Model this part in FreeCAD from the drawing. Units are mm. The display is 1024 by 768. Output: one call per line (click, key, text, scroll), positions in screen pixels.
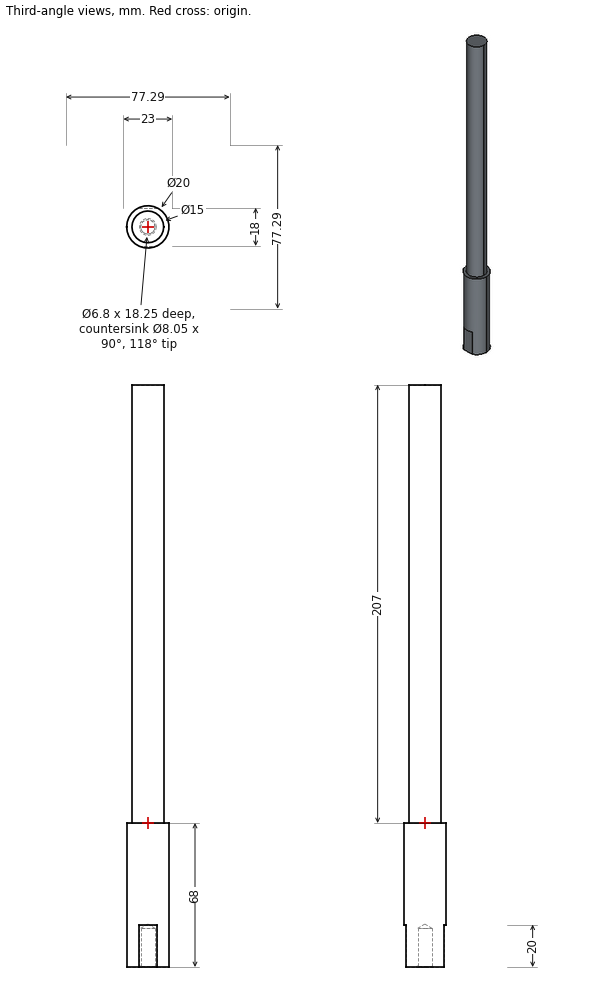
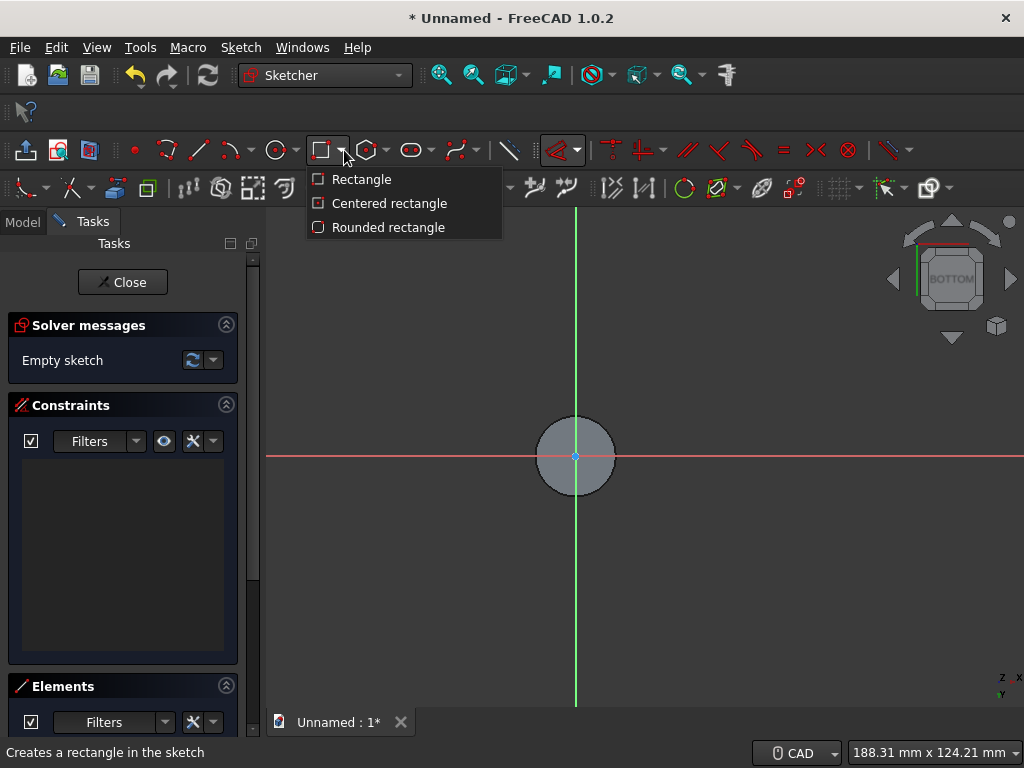
click(404, 203)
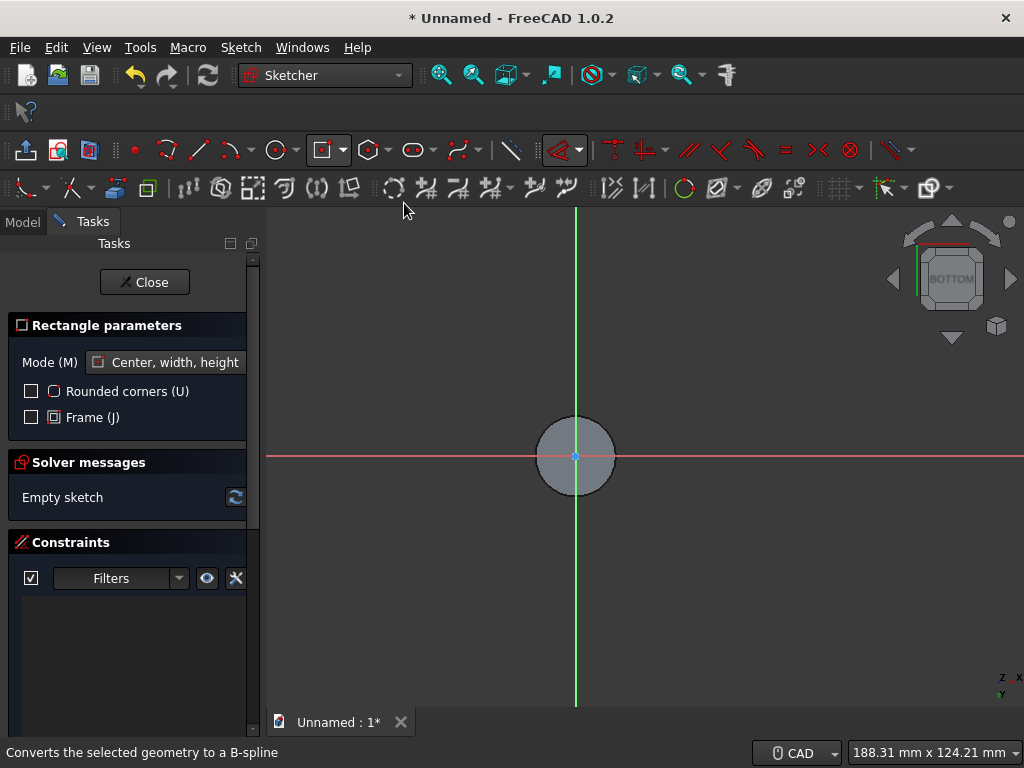
click(576, 456)
click(731, 301)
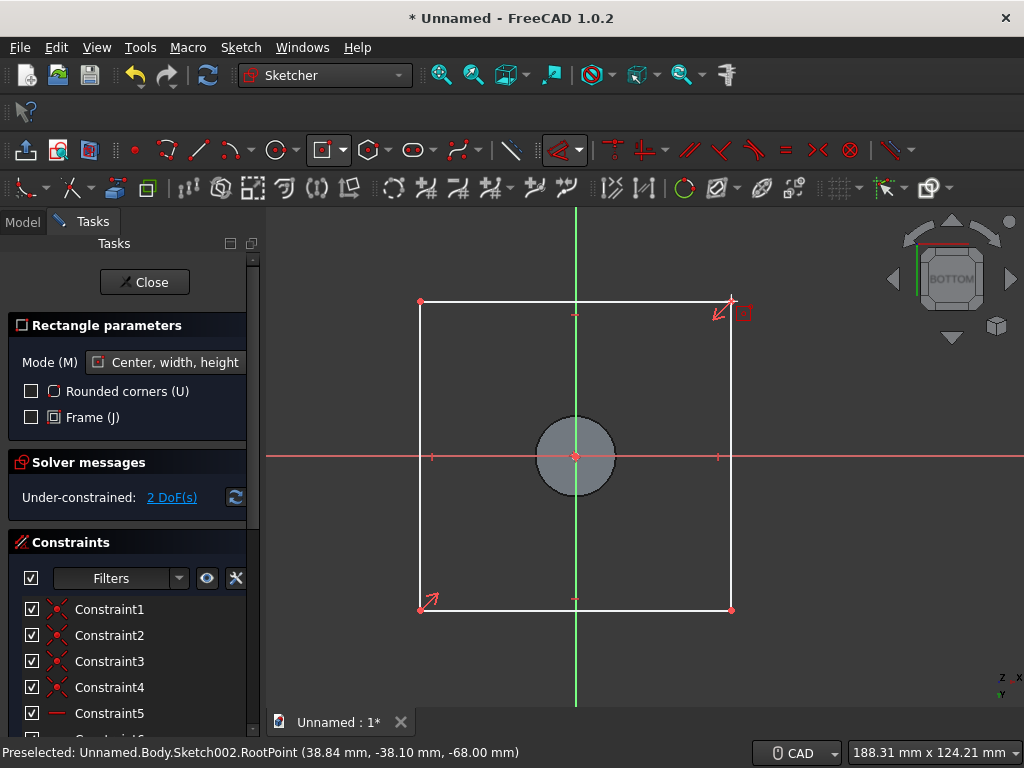
click(576, 456)
click(622, 420)
key(Escape)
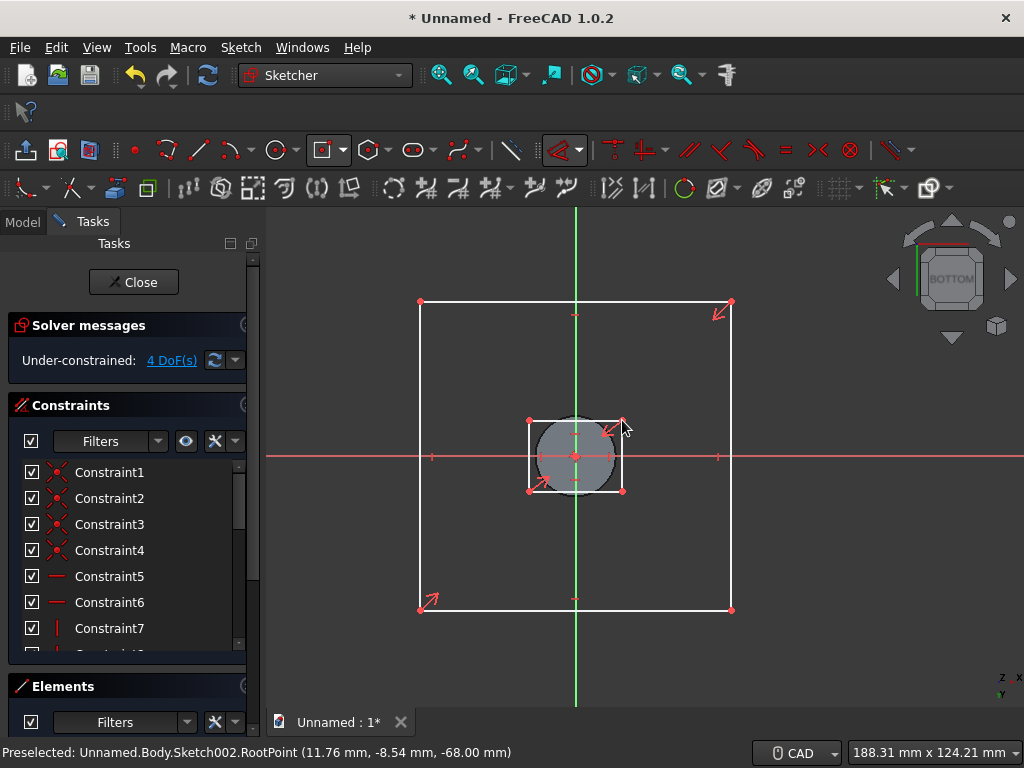
click(557, 492)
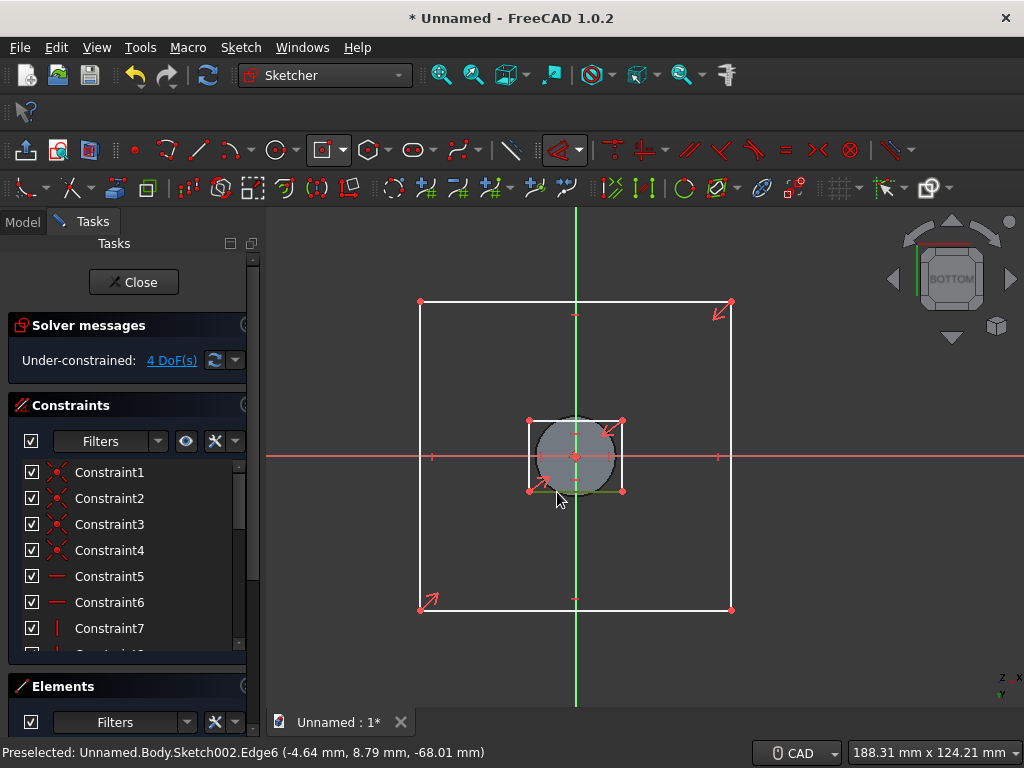
key(l)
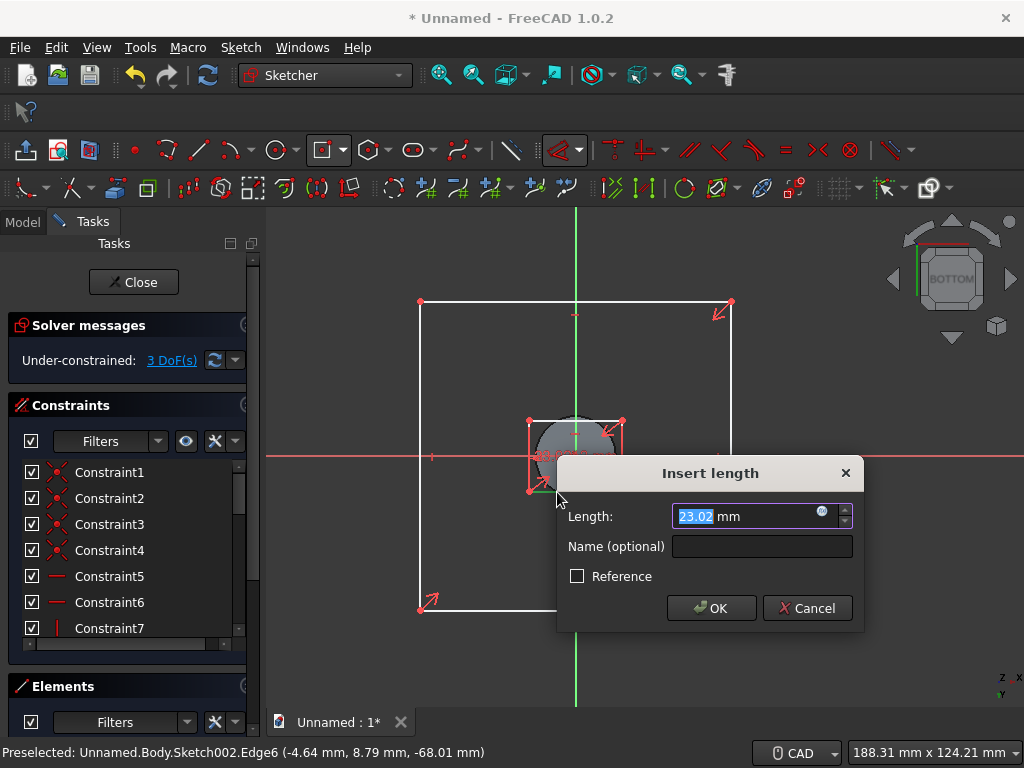
text(23)
key(Return)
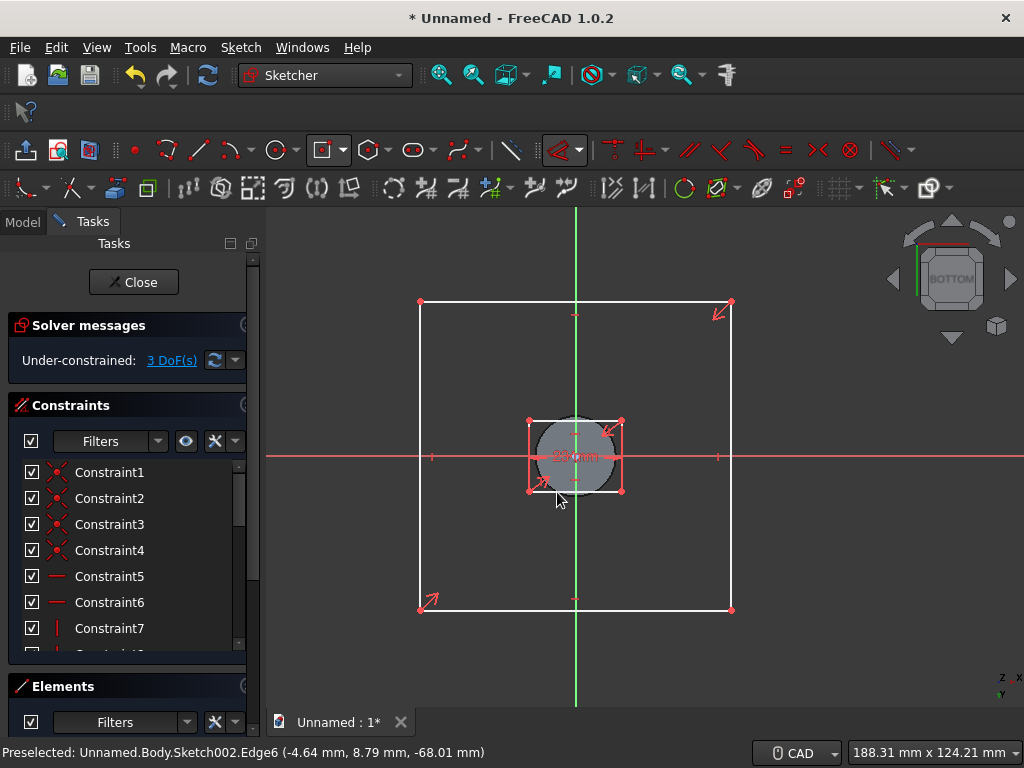
click(622, 471)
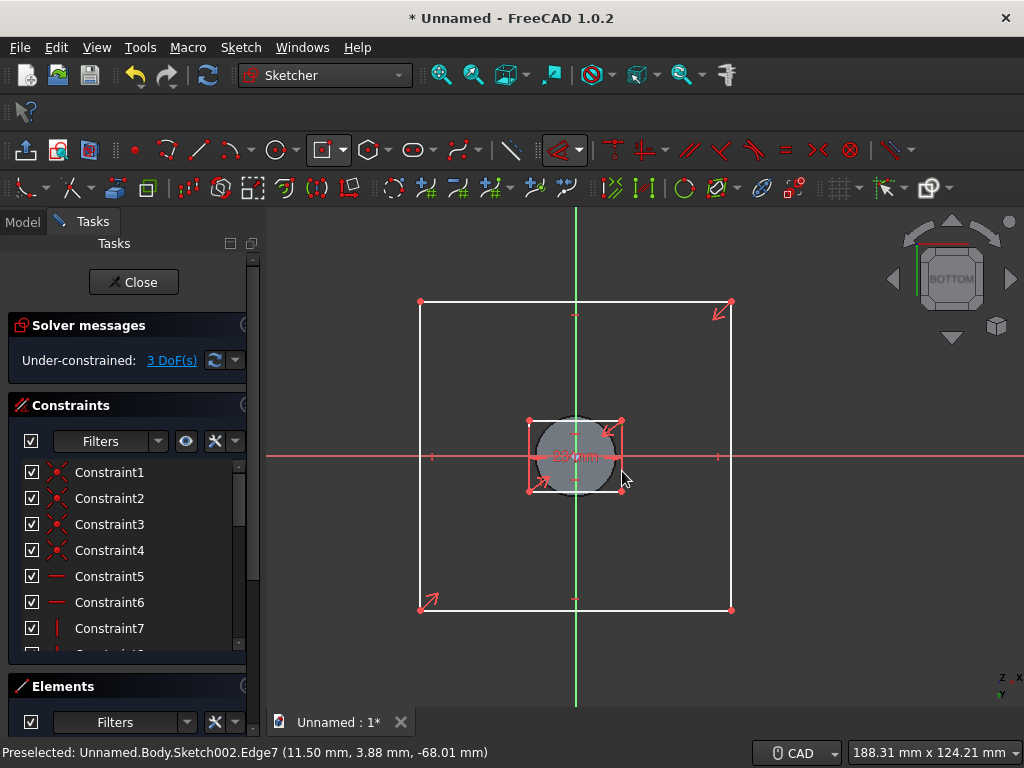
click(582, 150)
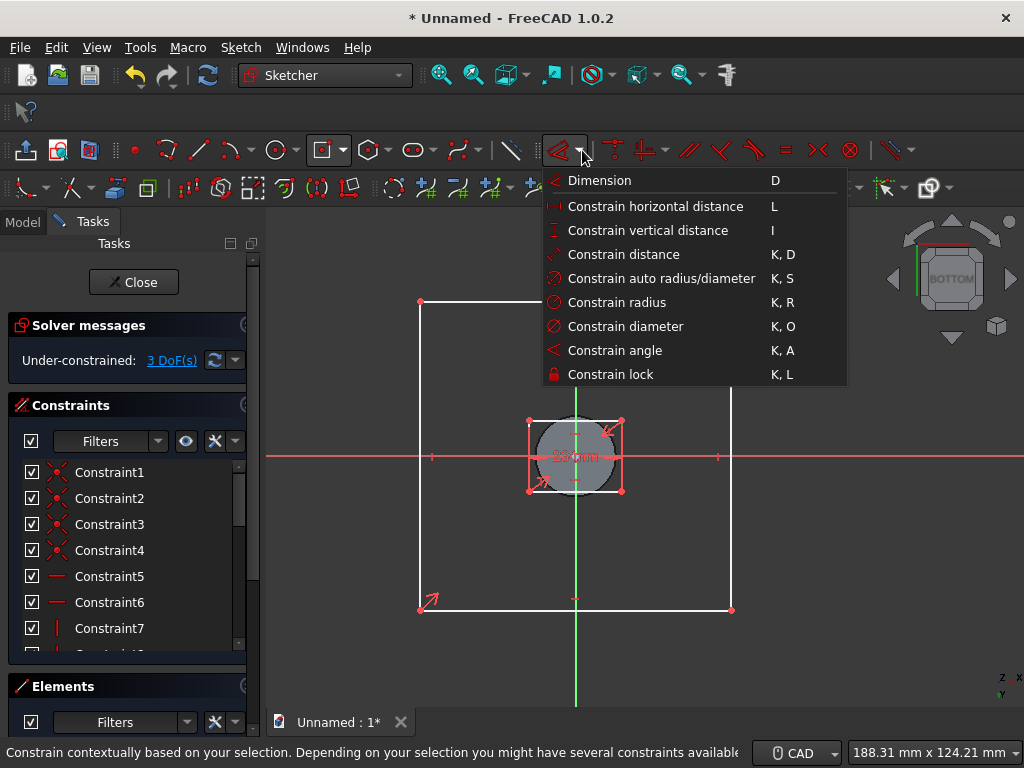
click(695, 230)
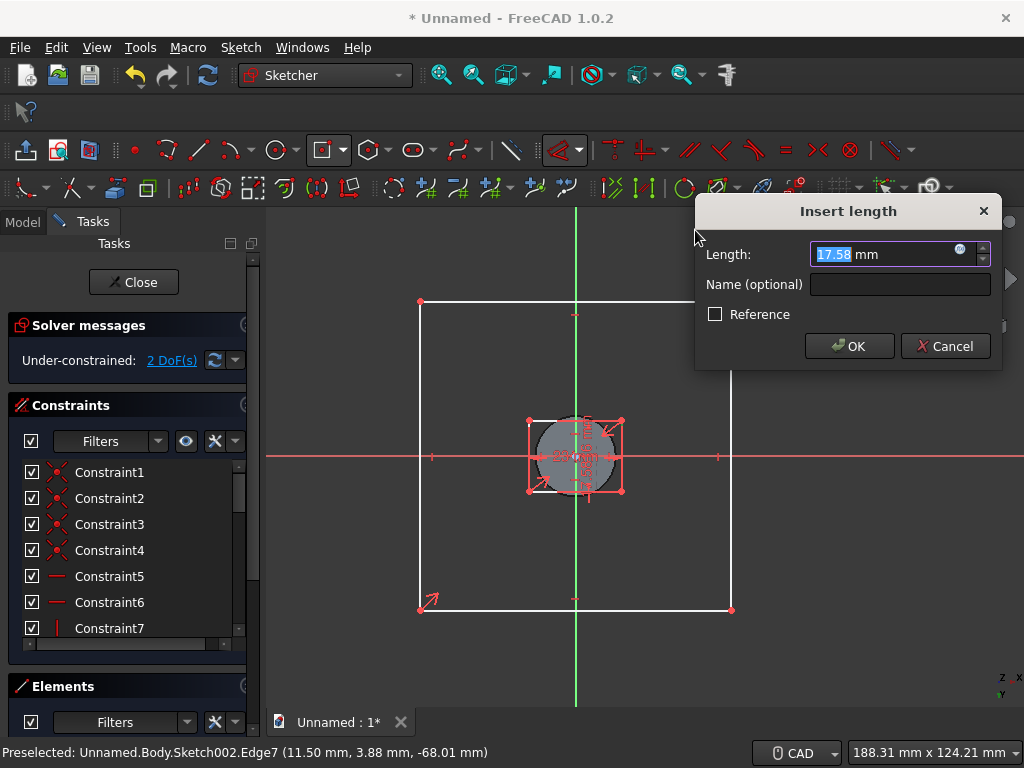
text(18)
key(Return)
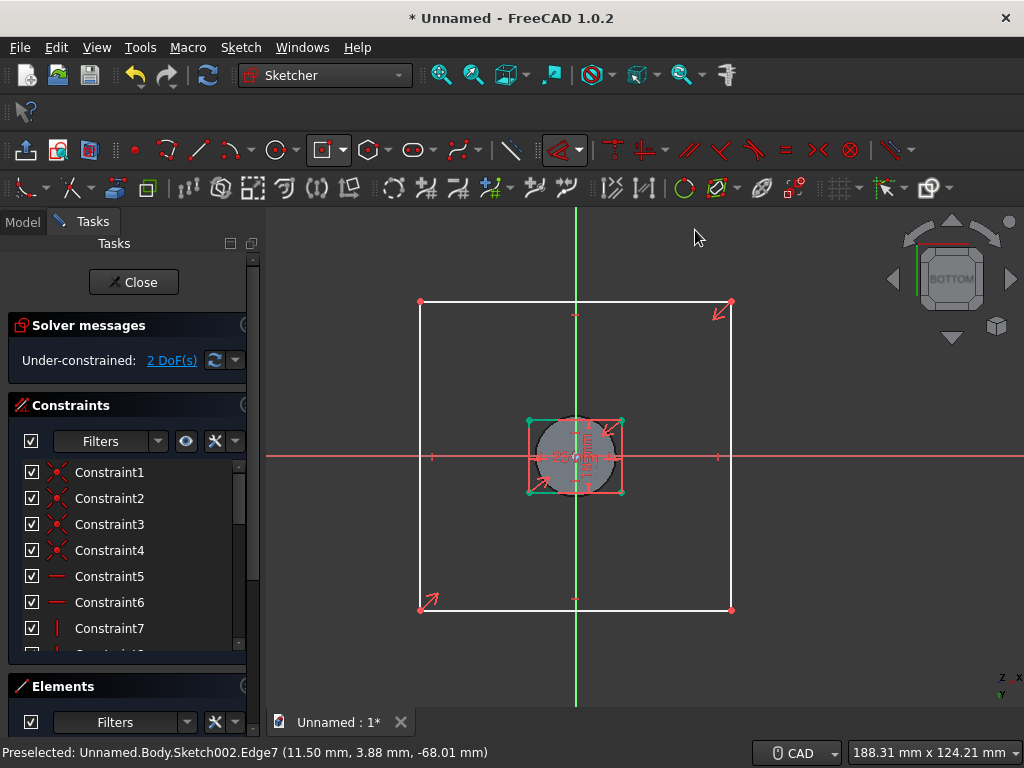
click(514, 611)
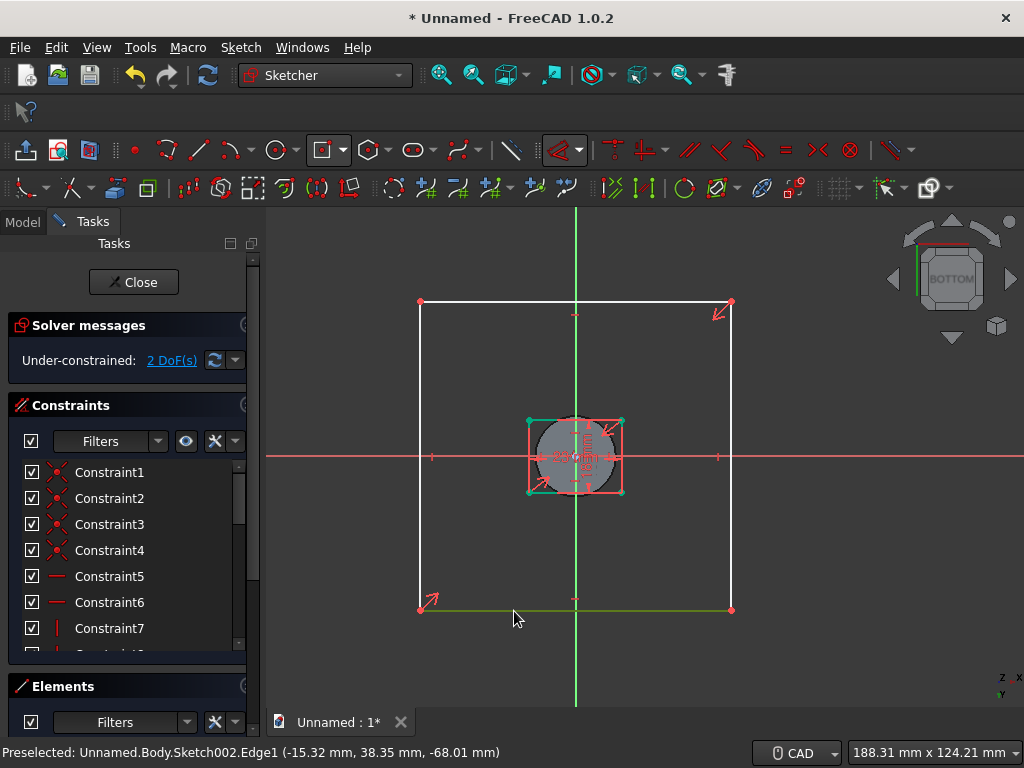
click(582, 150)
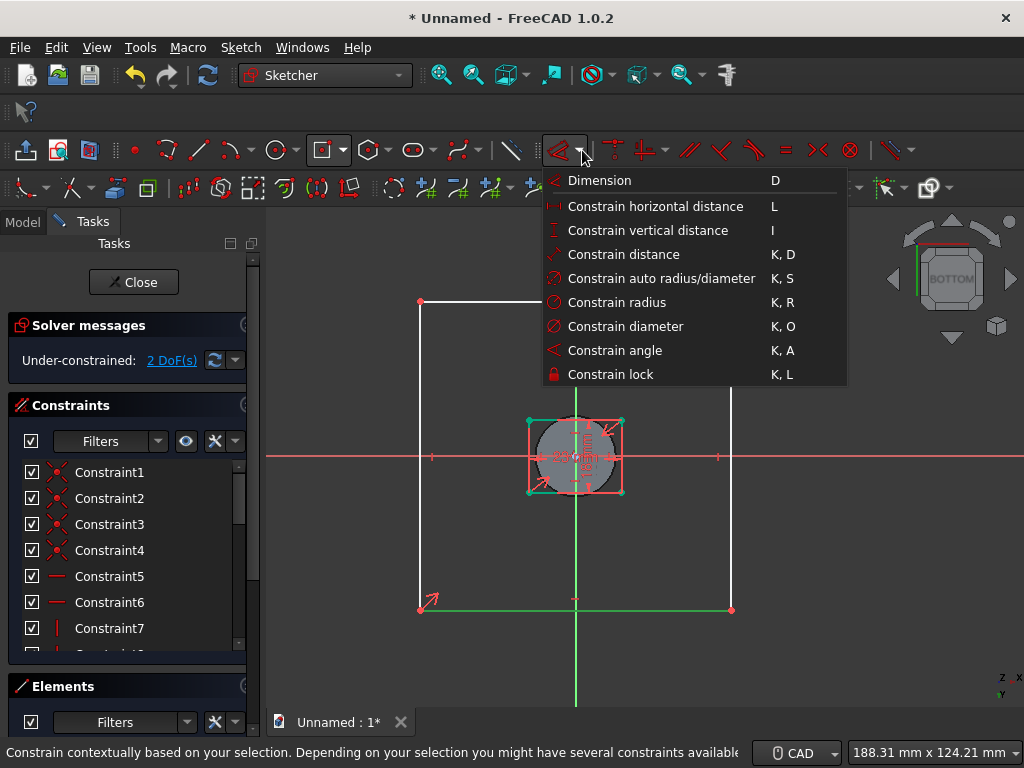
click(695, 206)